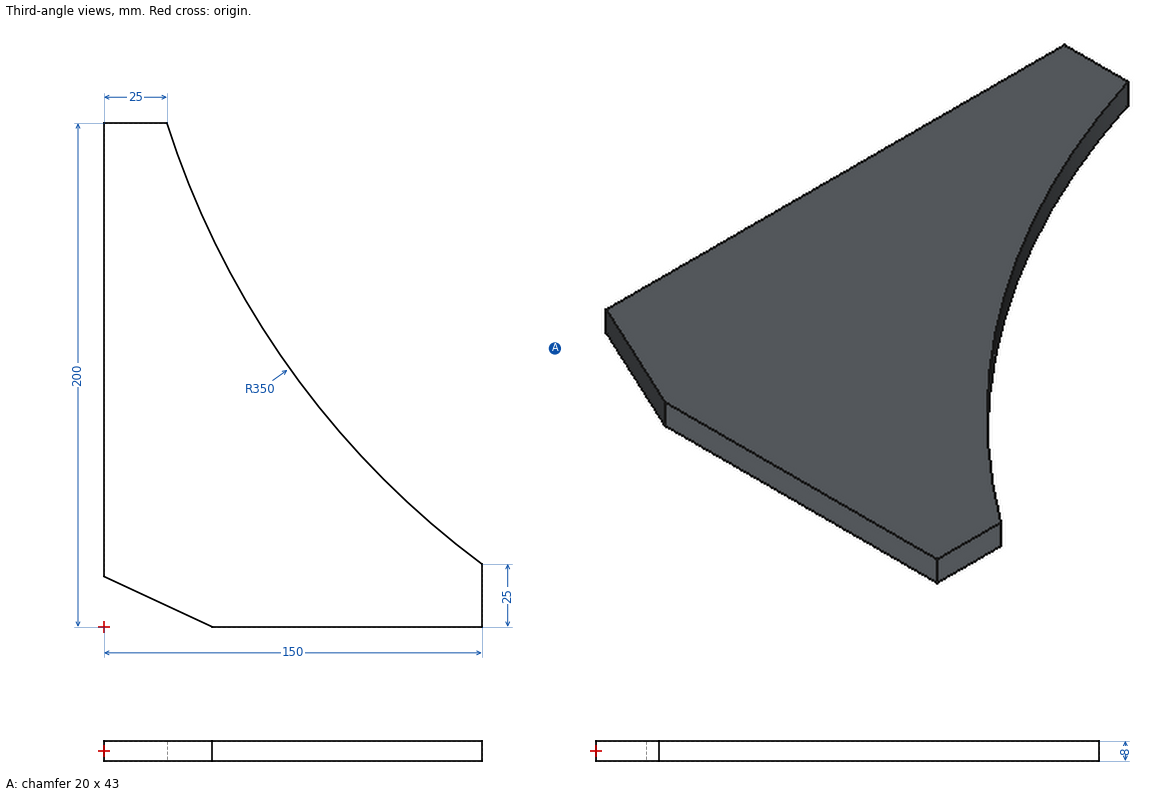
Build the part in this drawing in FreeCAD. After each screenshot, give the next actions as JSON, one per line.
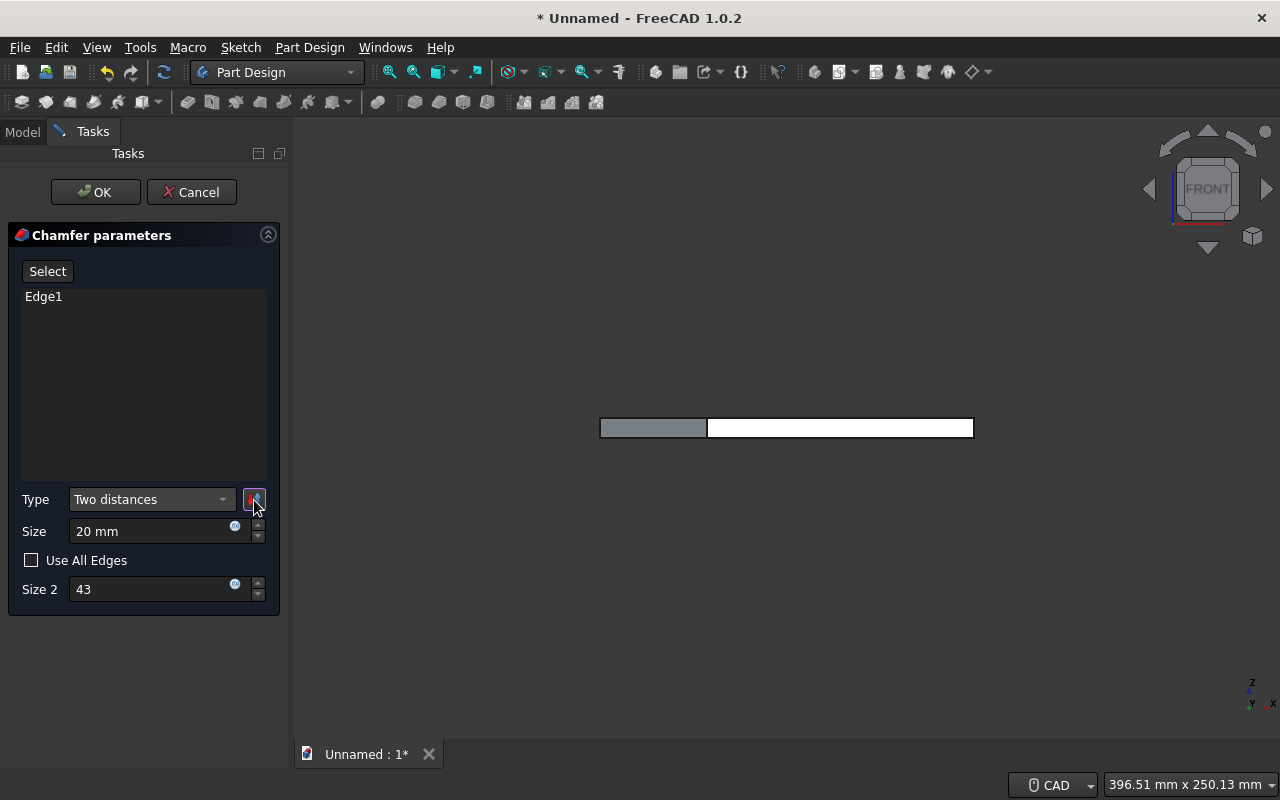
{"action": "left_click", "coordinate": [96, 192]}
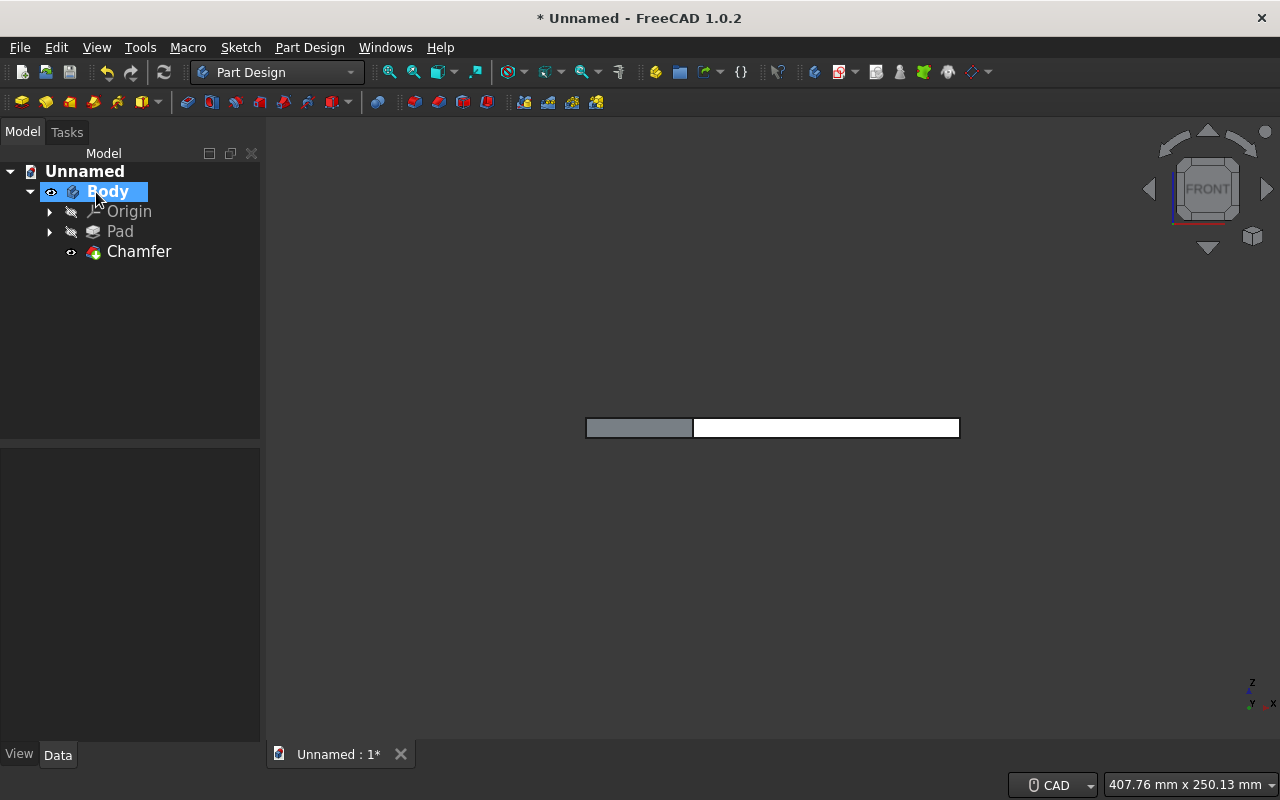
{"action": "key", "text": "v f"}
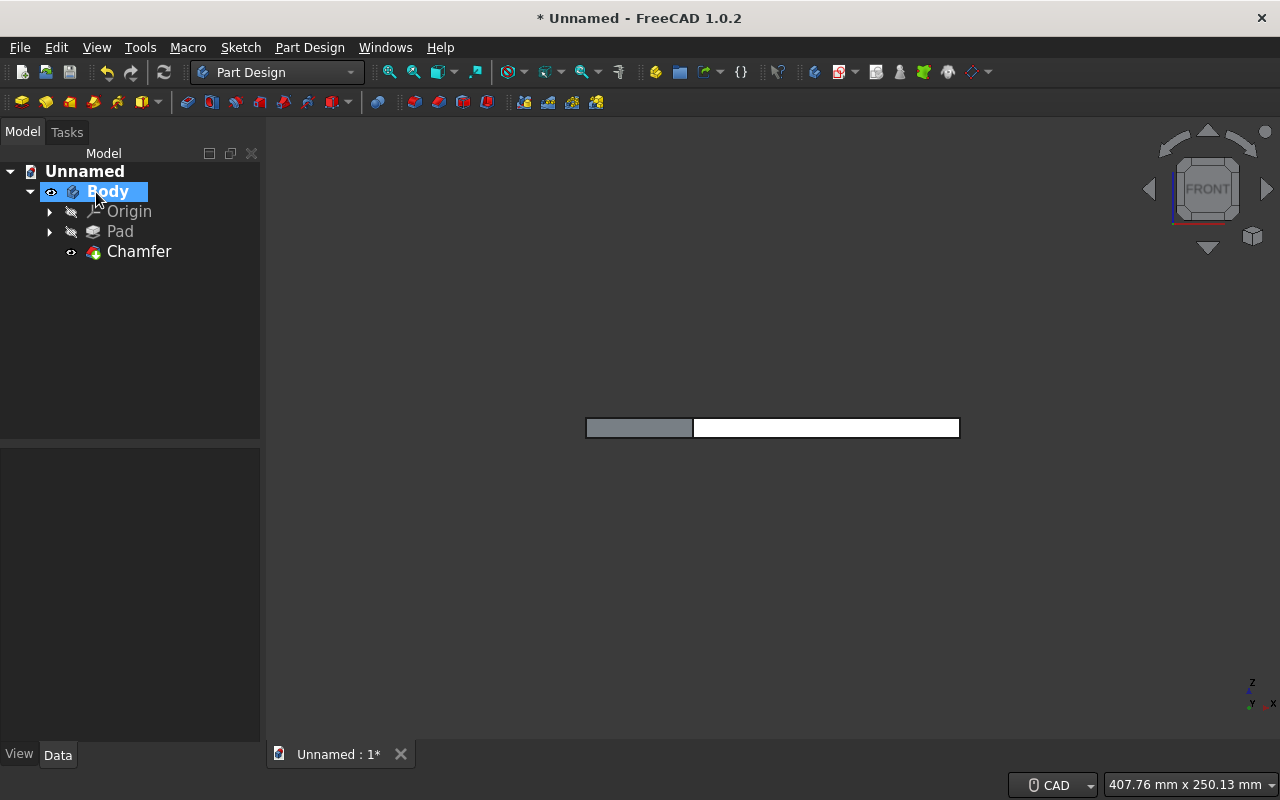
{"action": "key", "text": "0"}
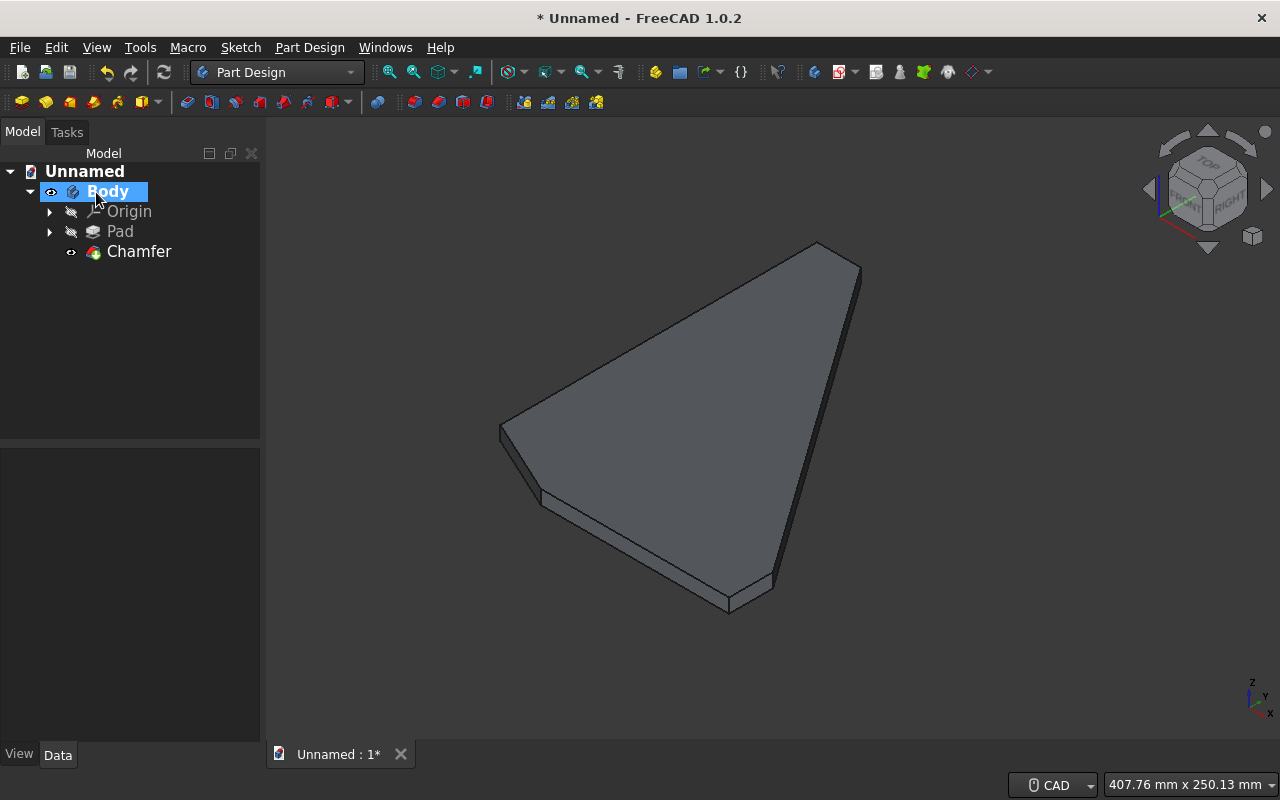
{"action": "left_click", "coordinate": [685, 426]}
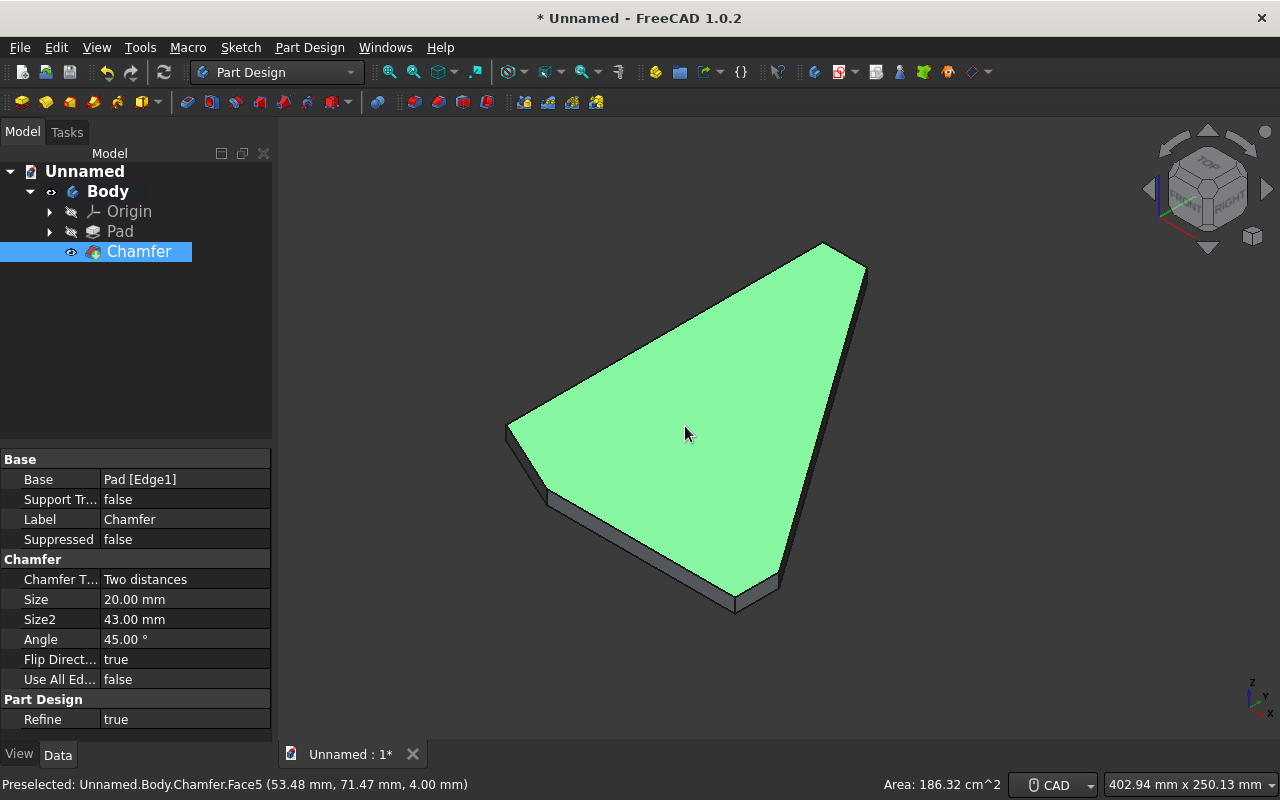
{"action": "left_click", "coordinate": [840, 72]}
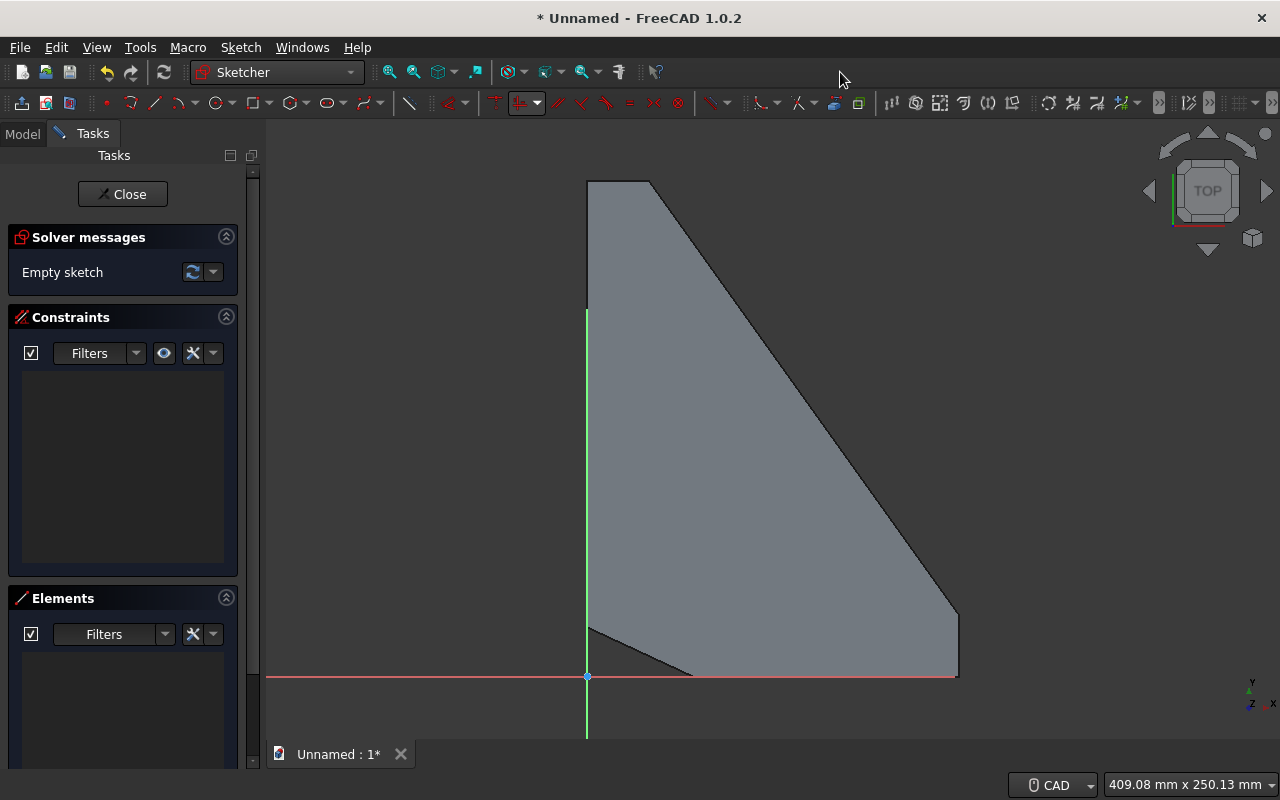
{"action": "key", "text": "g l"}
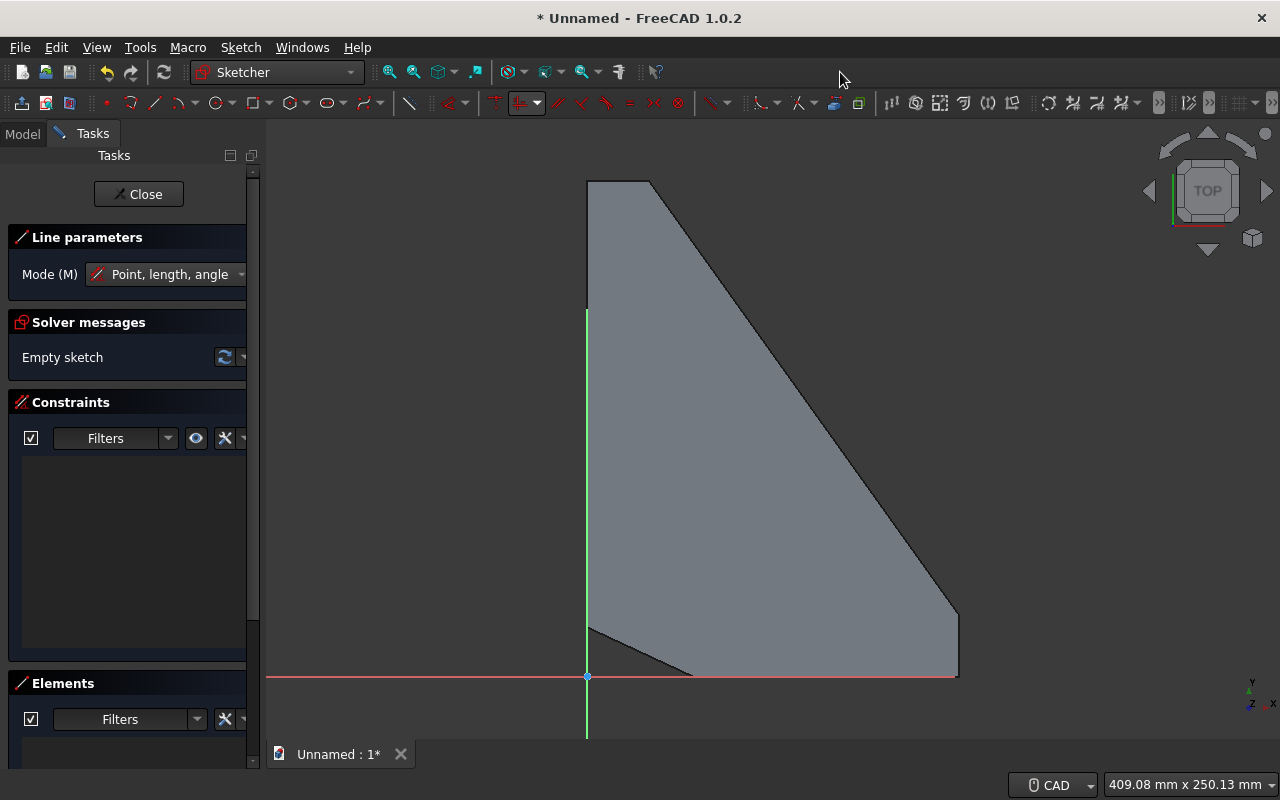
{"action": "left_click", "coordinate": [959, 615]}
{"action": "left_click", "coordinate": [649, 181]}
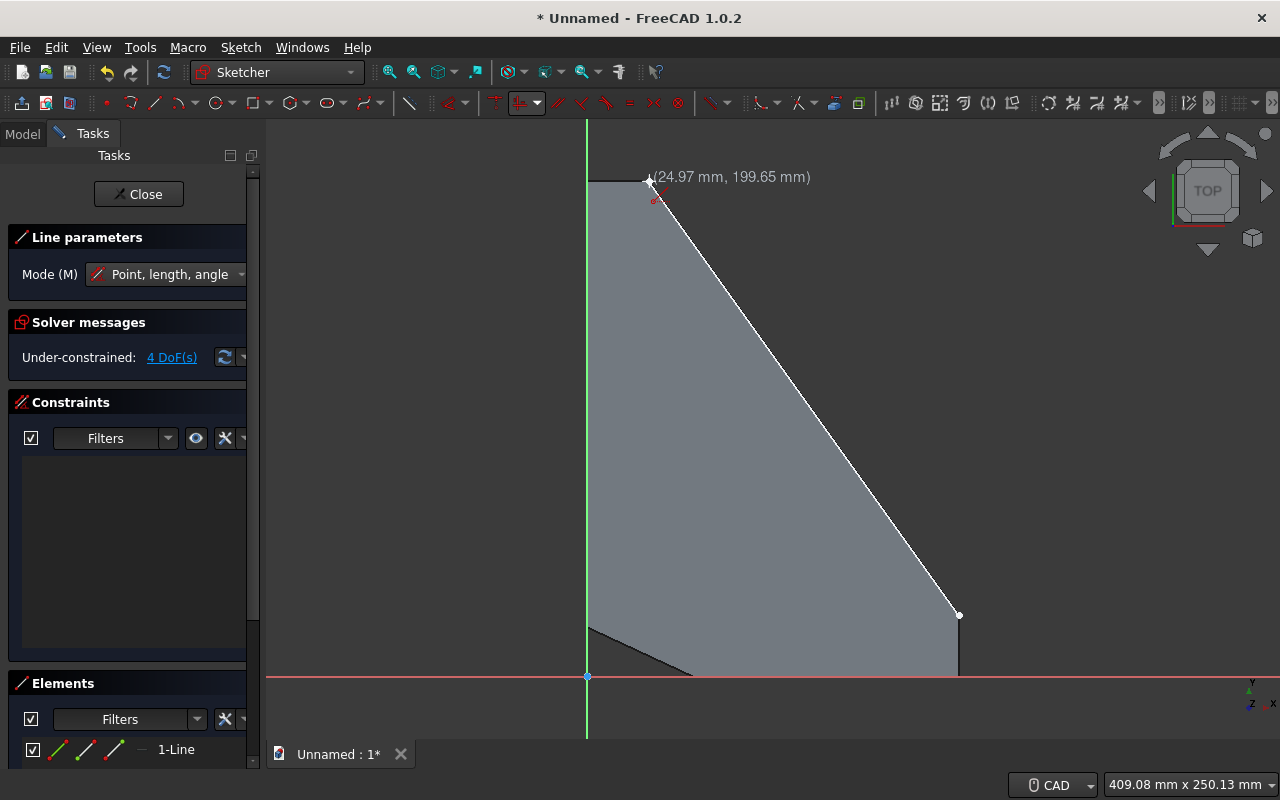
{"action": "key", "text": "g 3 a"}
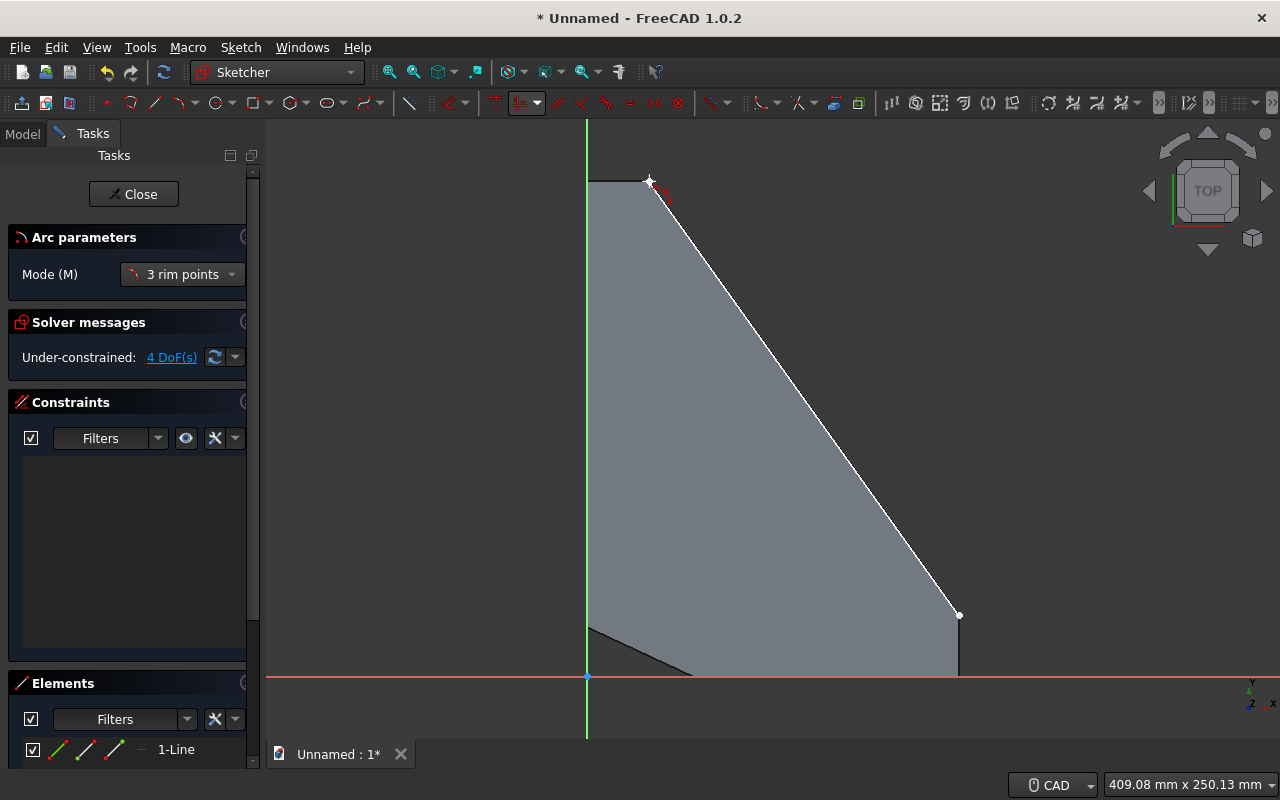
{"action": "left_click", "coordinate": [649, 182]}
{"action": "left_click", "coordinate": [959, 616]}
{"action": "left_click", "coordinate": [770, 422]}
{"action": "key", "text": "Escape"}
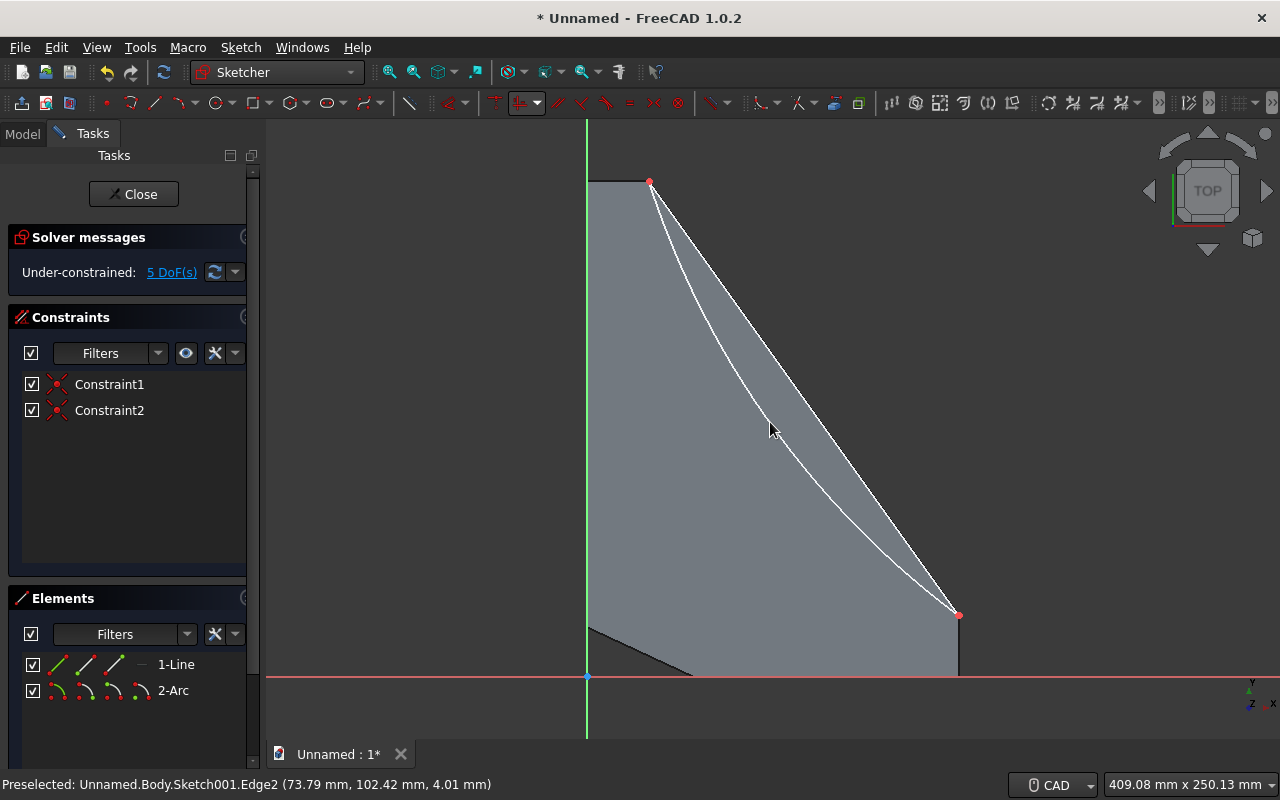
{"action": "key", "text": "d"}